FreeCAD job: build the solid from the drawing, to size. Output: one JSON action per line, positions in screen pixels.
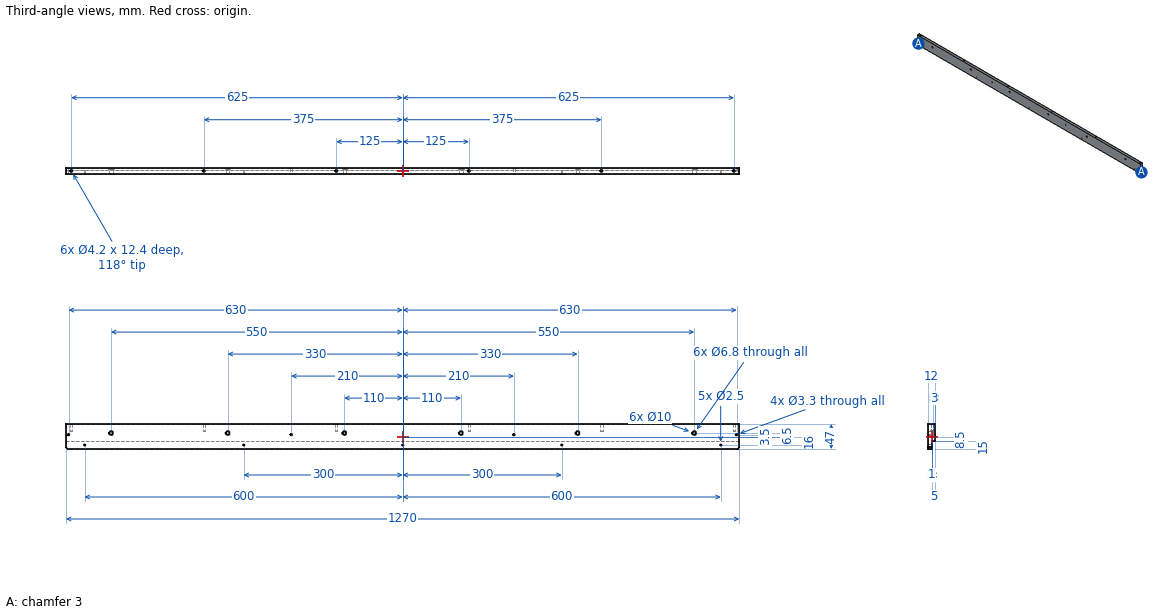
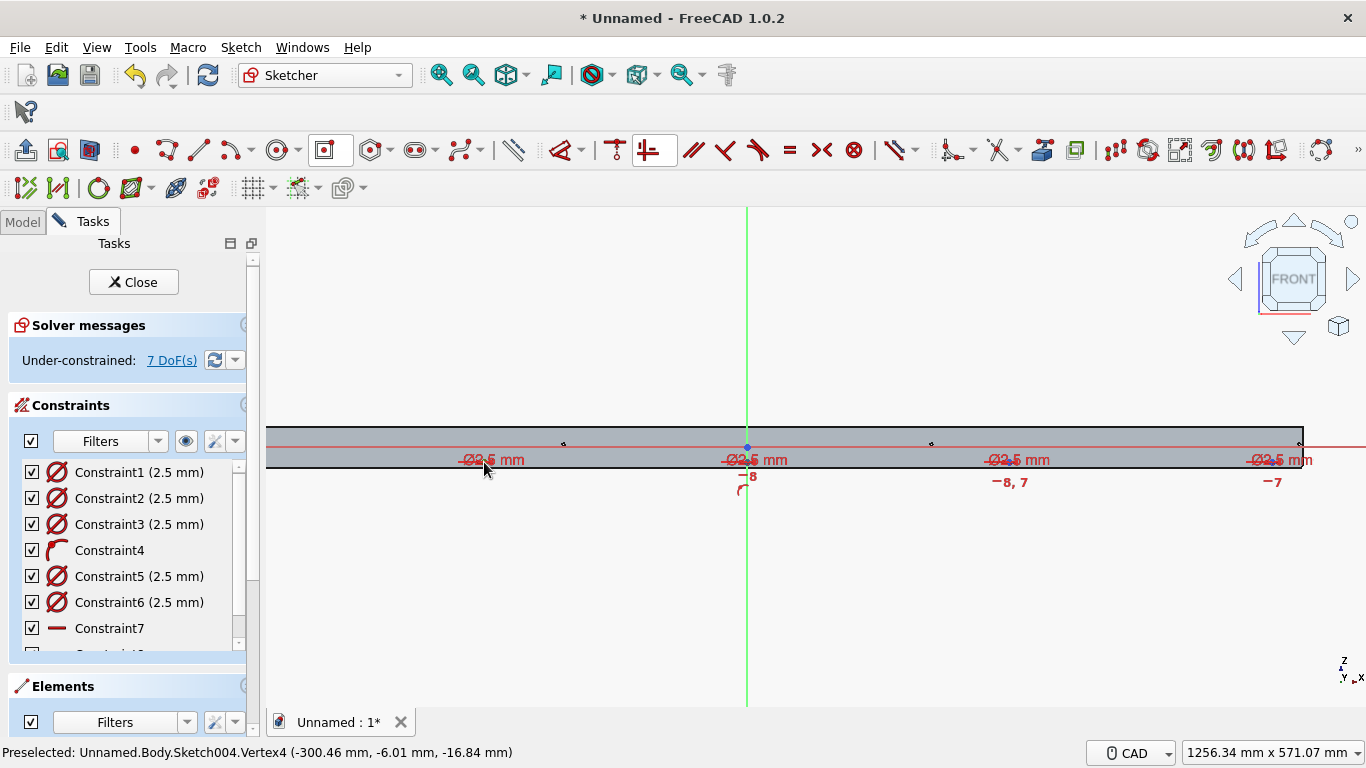
{"action": "key", "text": "h"}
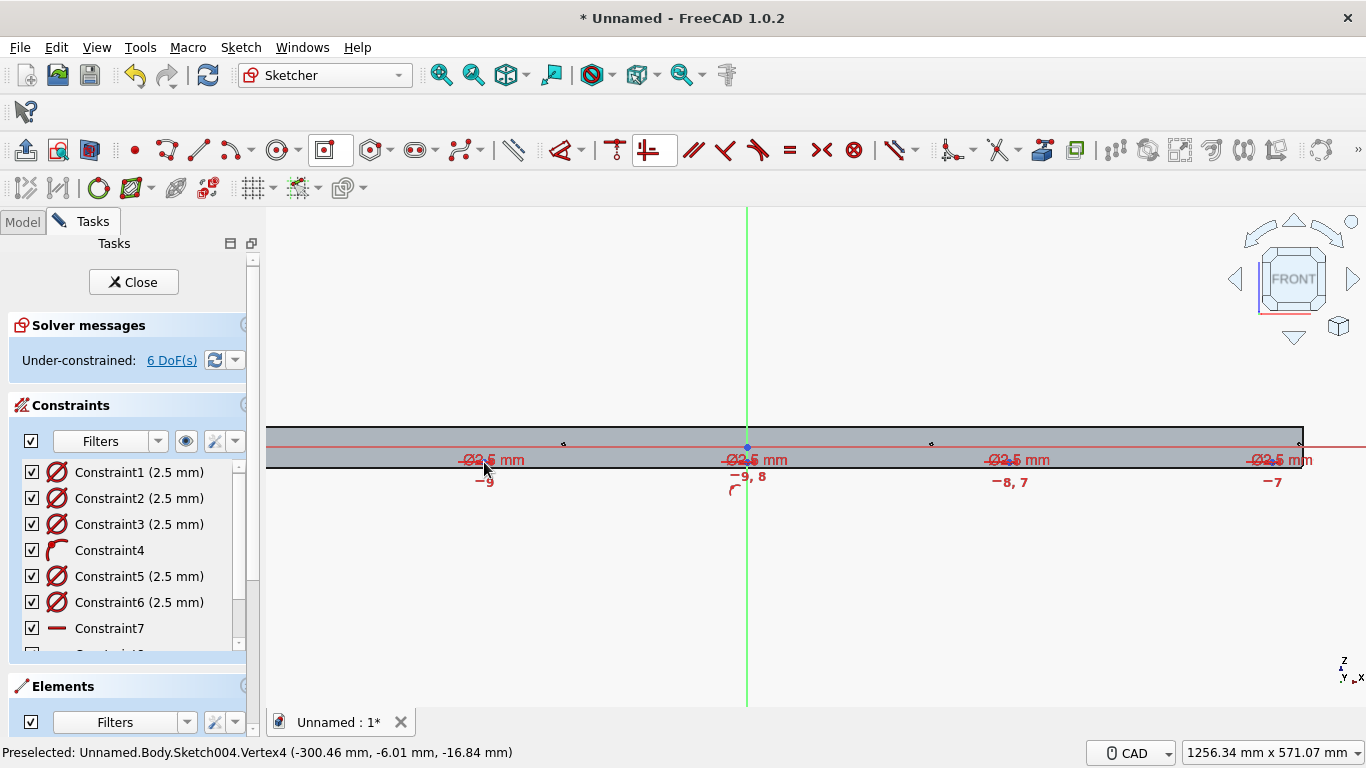
{"action": "left_click", "coordinate": [484, 462]}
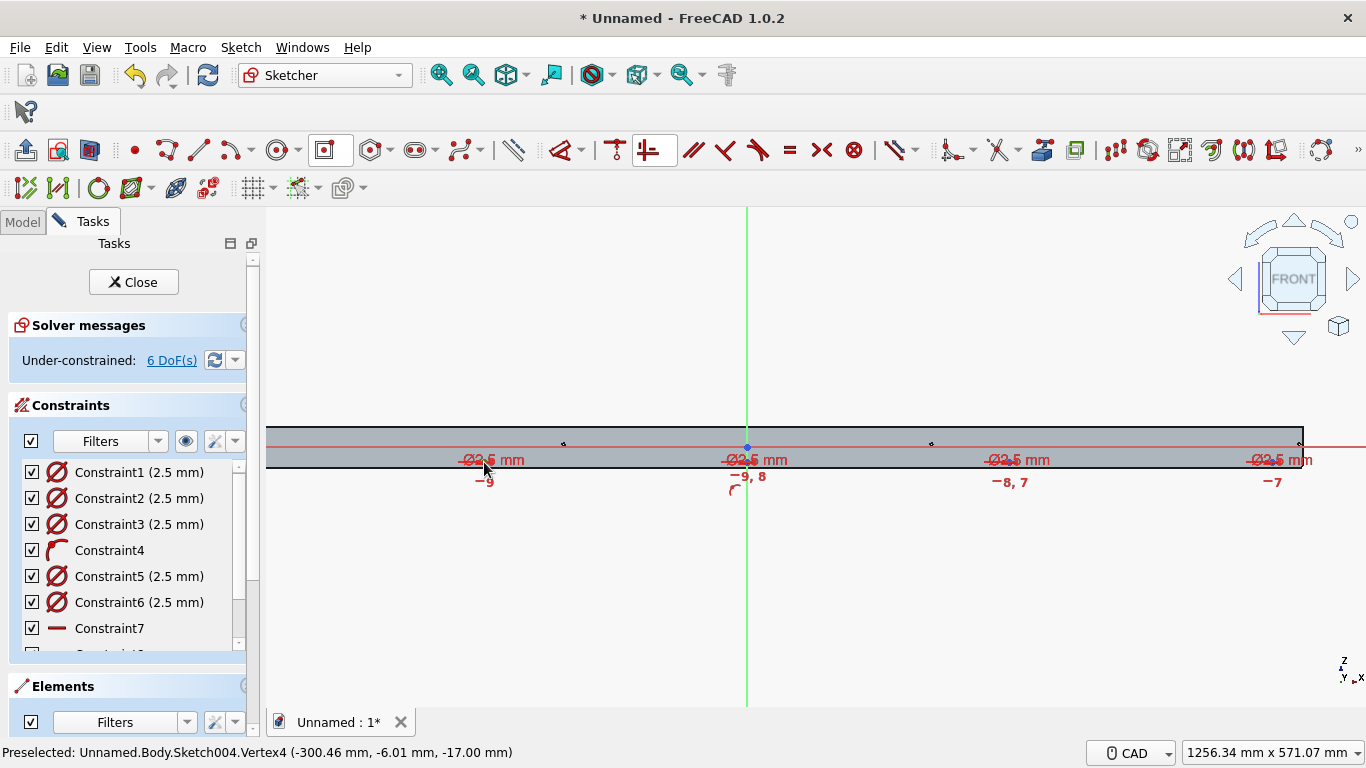
{"action": "scroll", "coordinate": [748, 461], "scroll_direction": "down", "scroll_amount": 2}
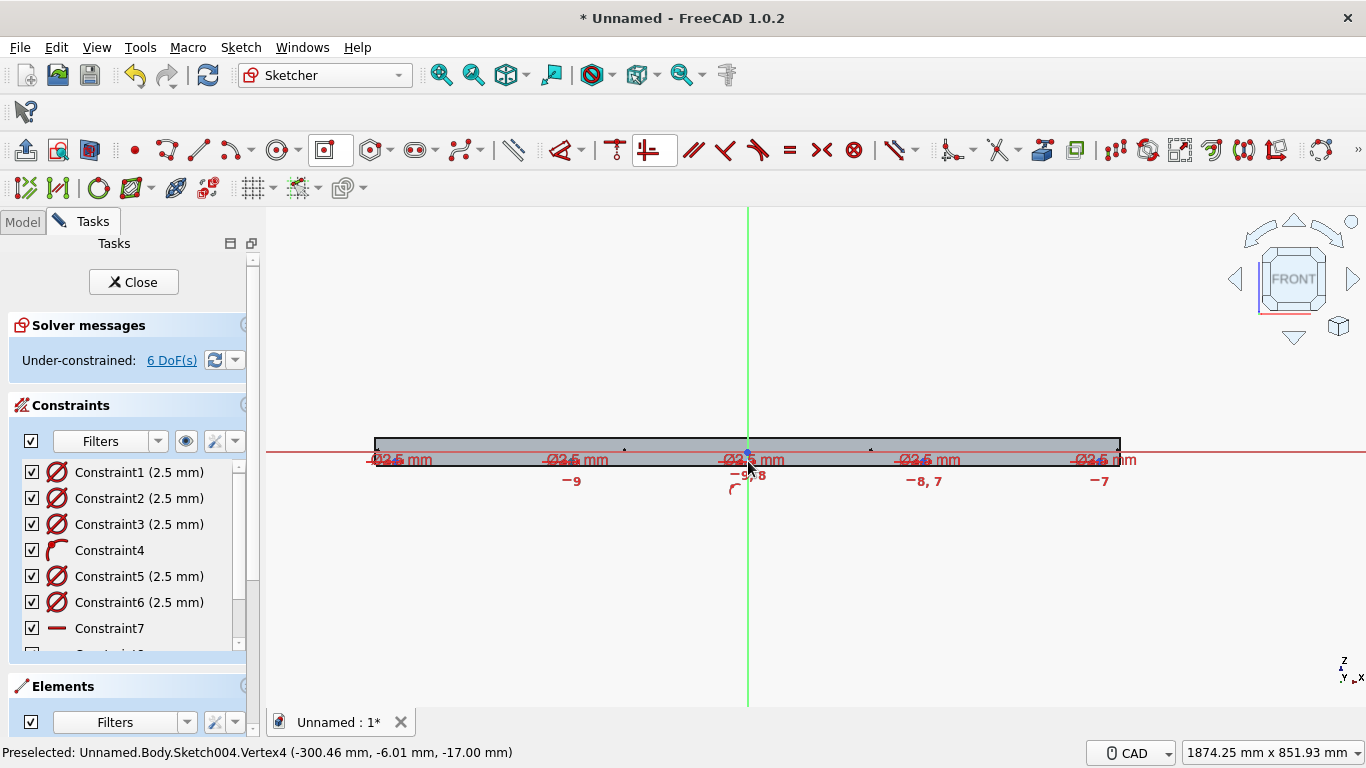
{"action": "left_click", "coordinate": [395, 462]}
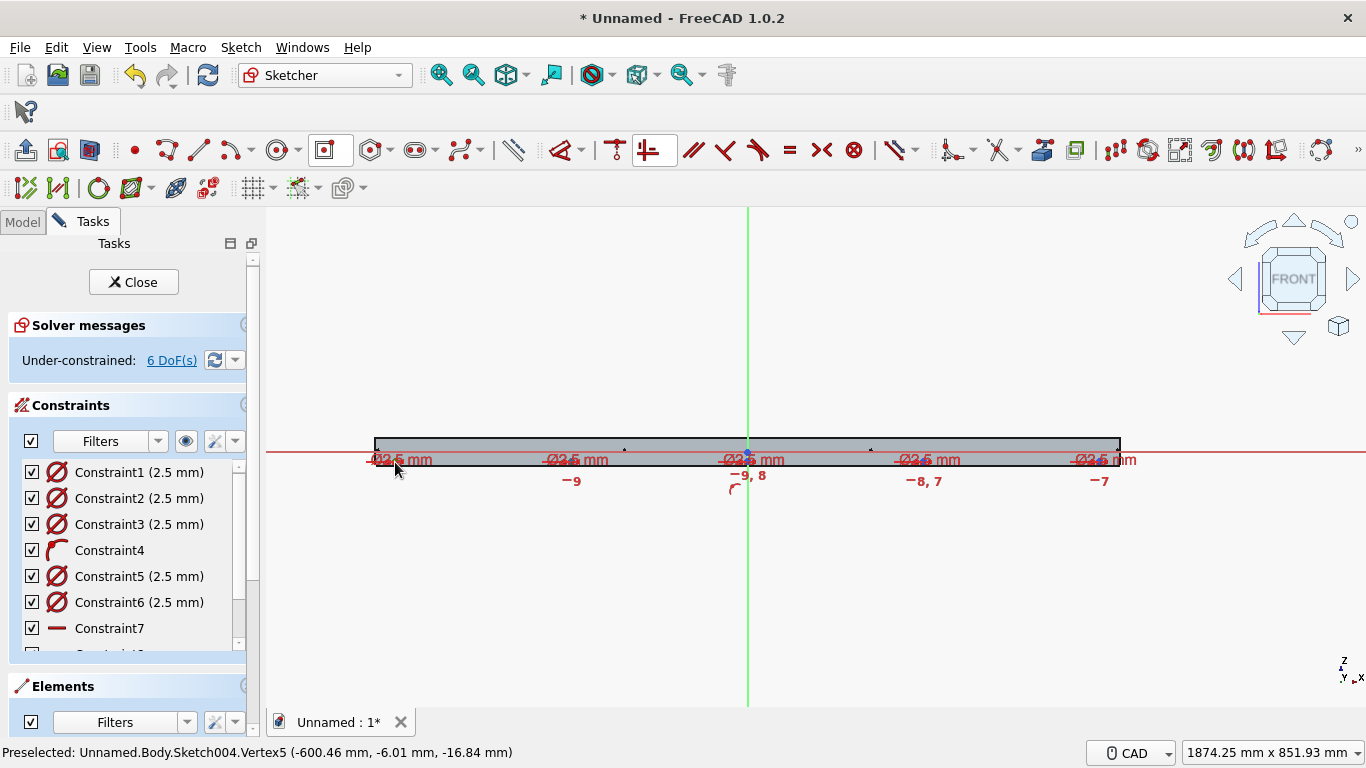
{"action": "key", "text": "h"}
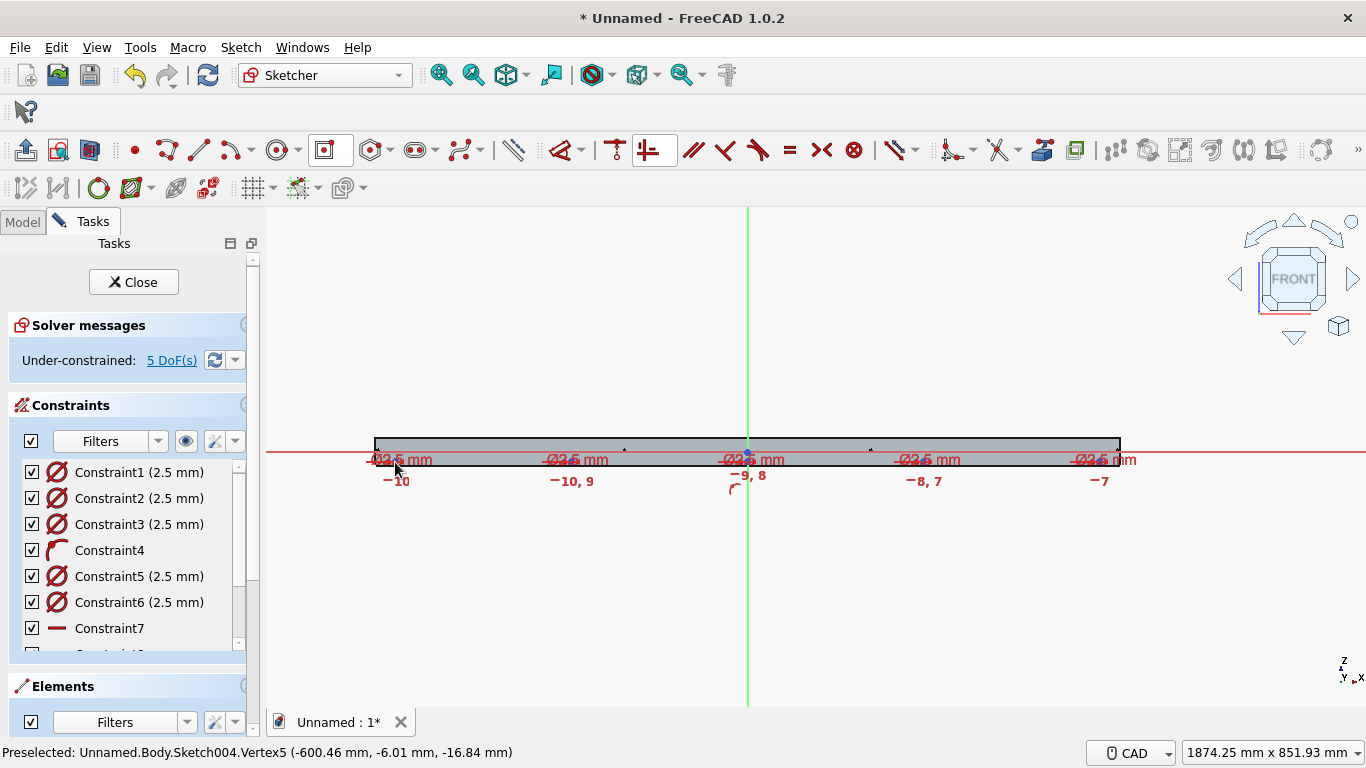
{"action": "left_click", "coordinate": [560, 150]}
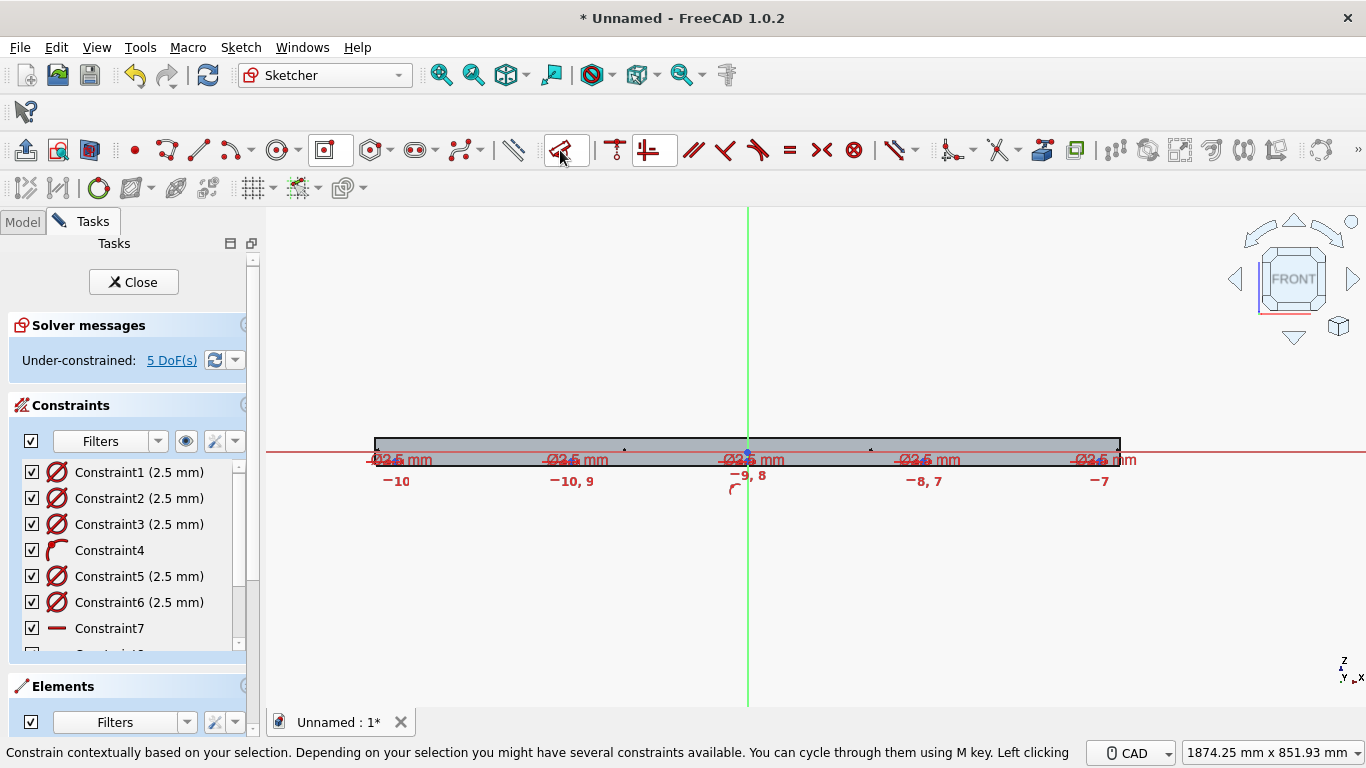
{"action": "scroll", "coordinate": [1100, 462], "scroll_direction": "up", "scroll_amount": 8}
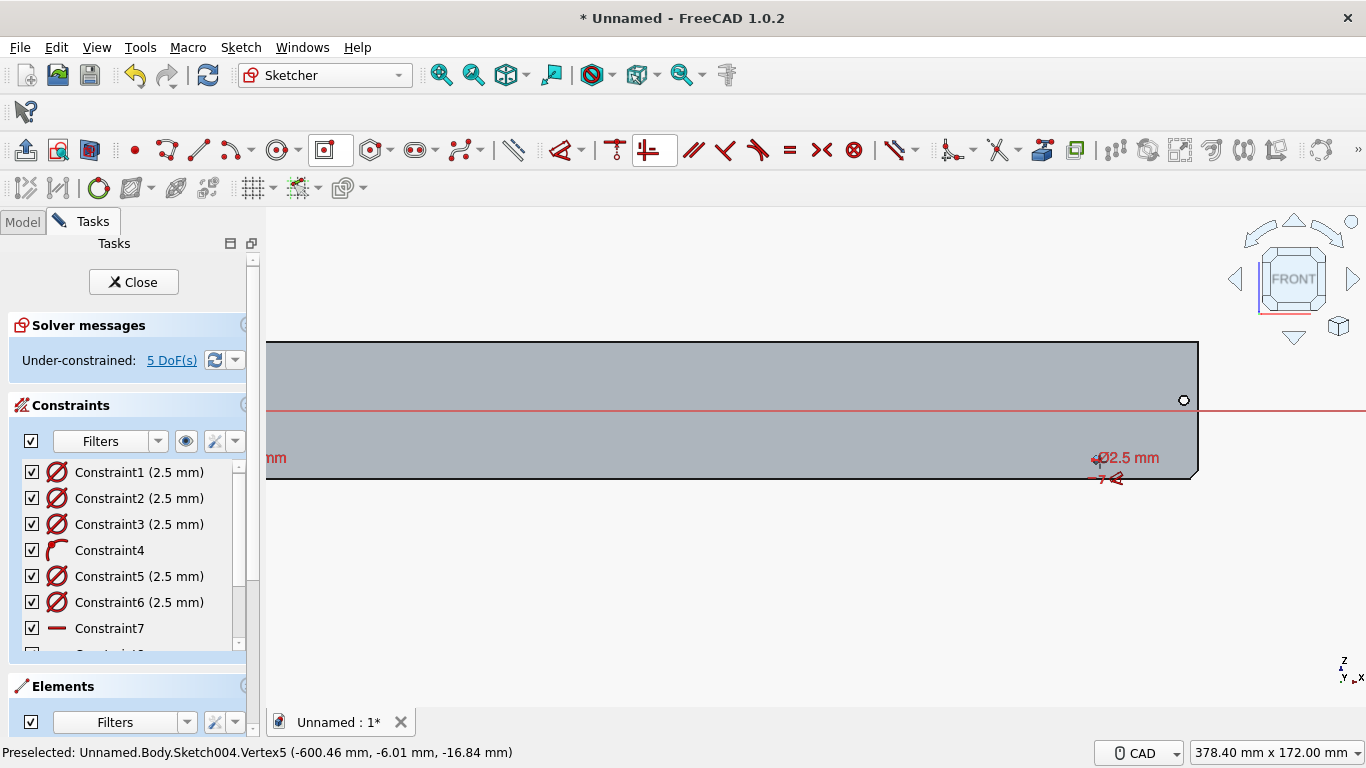
{"action": "left_click", "coordinate": [1096, 460]}
{"action": "left_click", "coordinate": [1130, 435]}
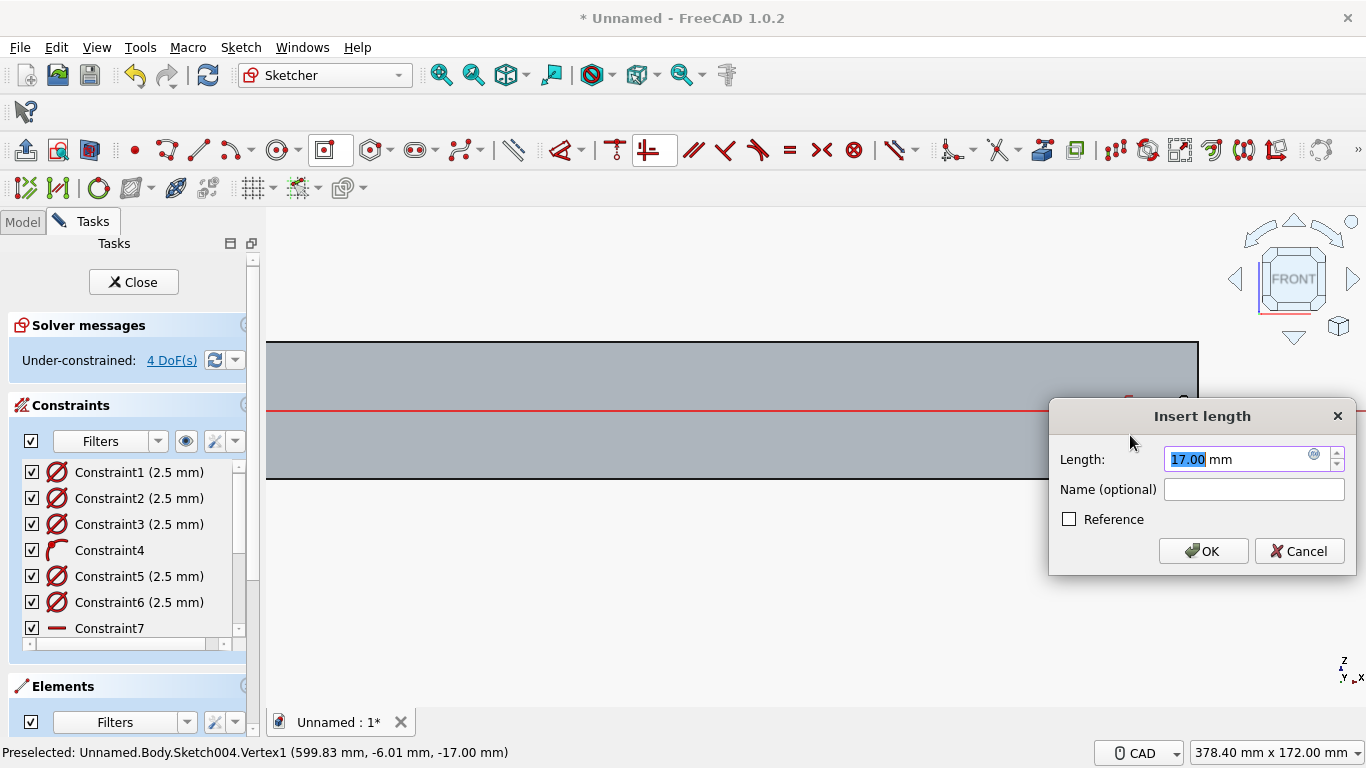
{"action": "type", "text": "16"}
{"action": "key", "text": "Return"}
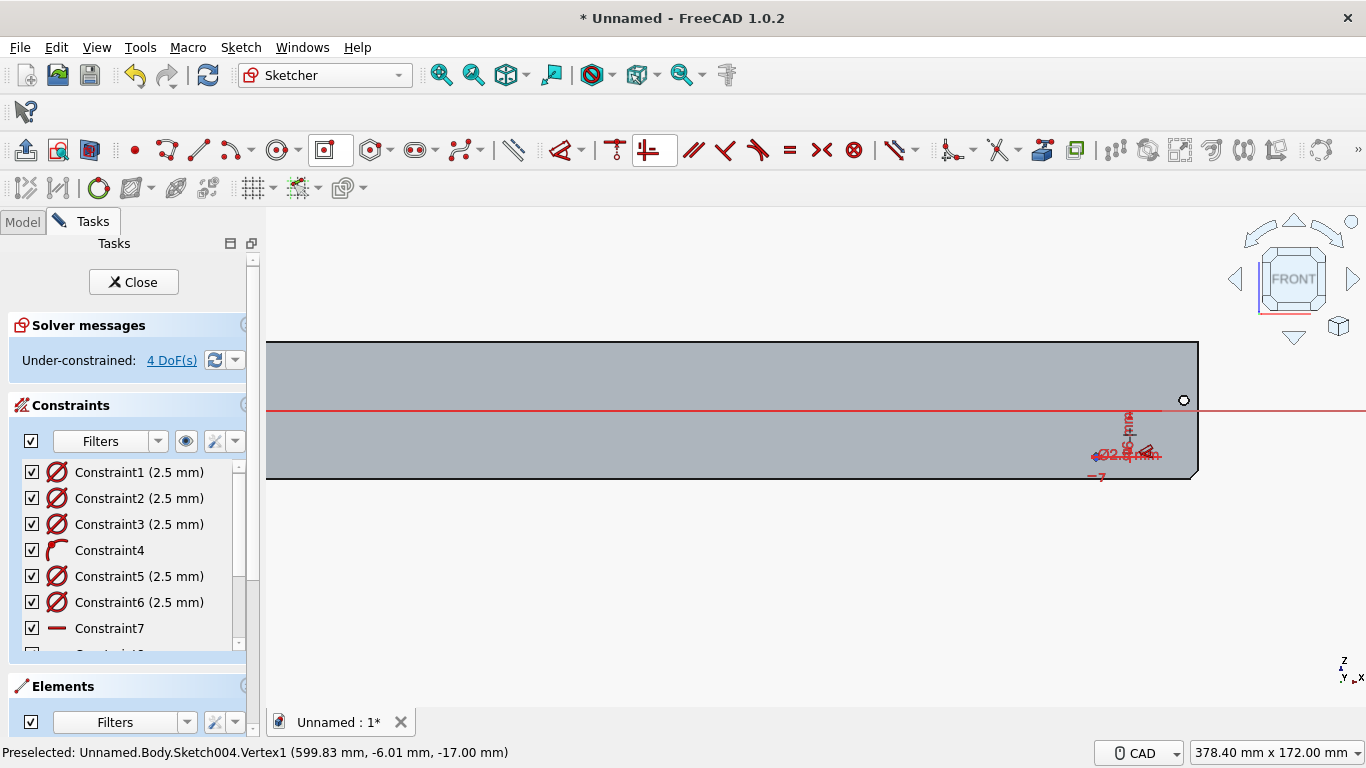
{"action": "scroll", "coordinate": [1100, 462], "scroll_direction": "down", "scroll_amount": 8}